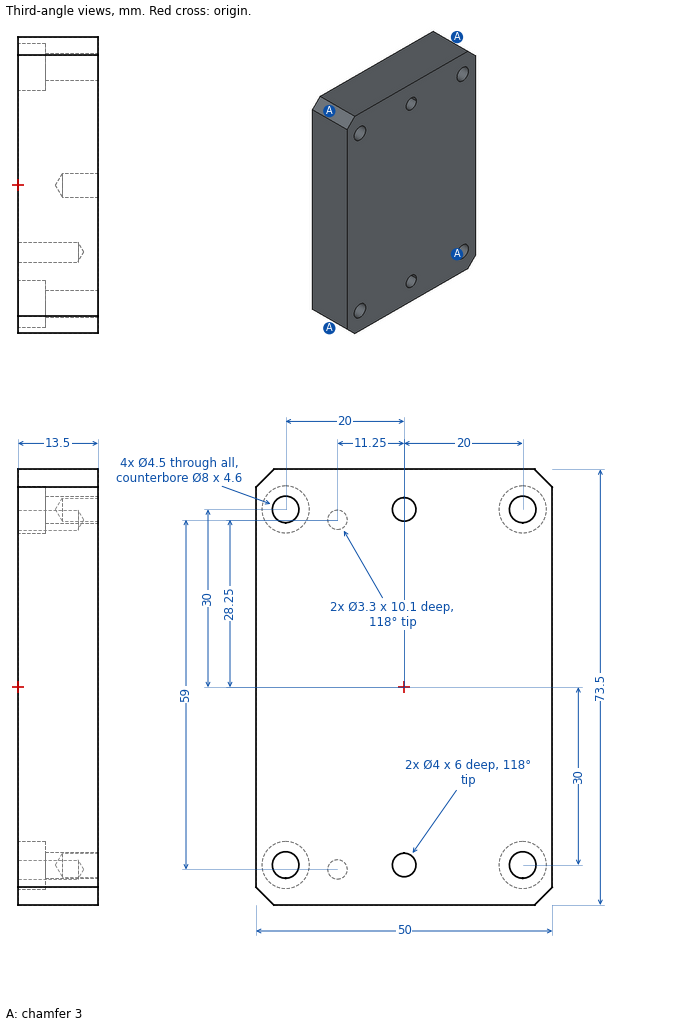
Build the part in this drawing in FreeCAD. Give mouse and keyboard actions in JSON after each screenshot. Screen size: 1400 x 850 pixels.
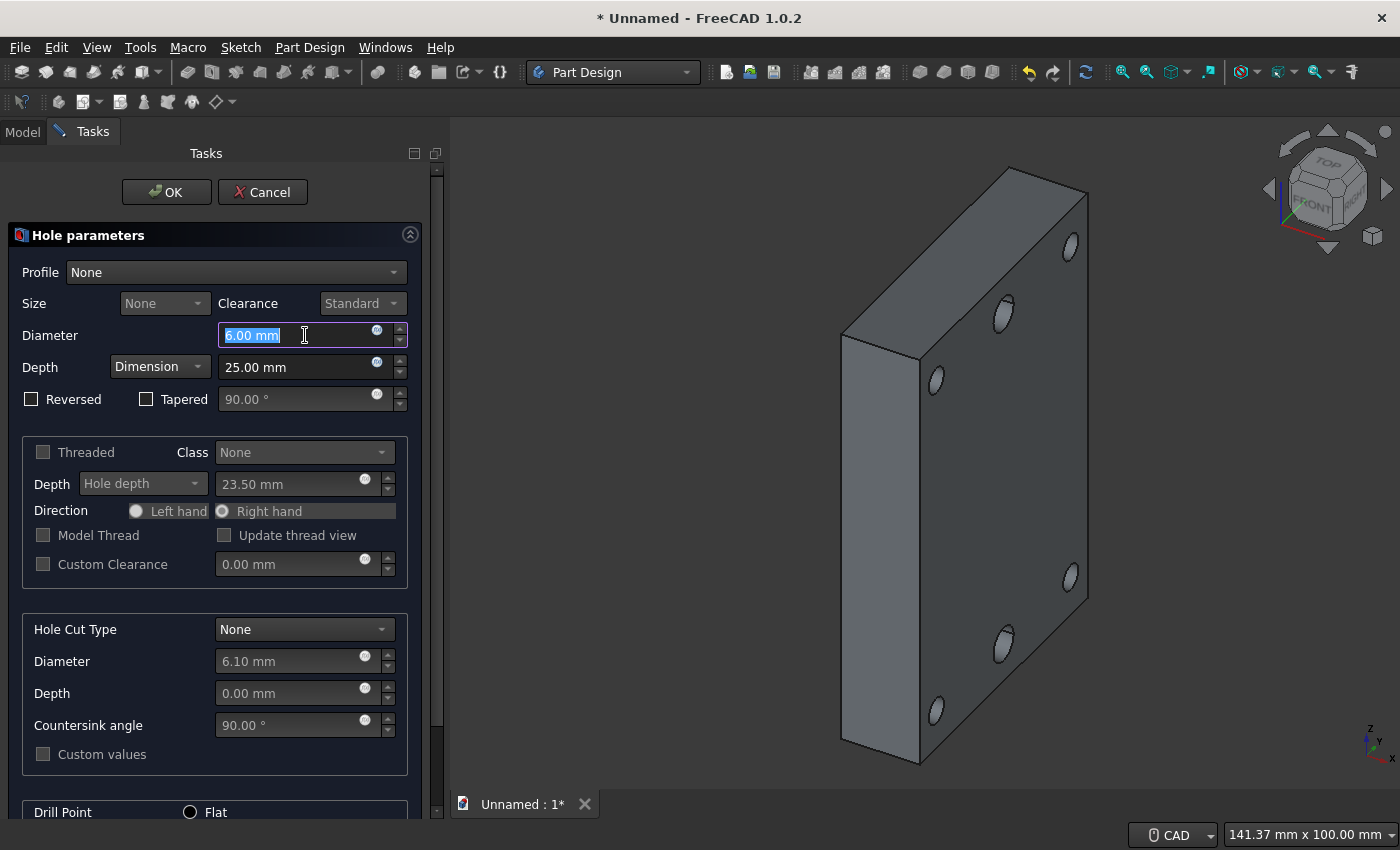
{"action": "type", "text": "4"}
{"action": "key", "text": "Tab"}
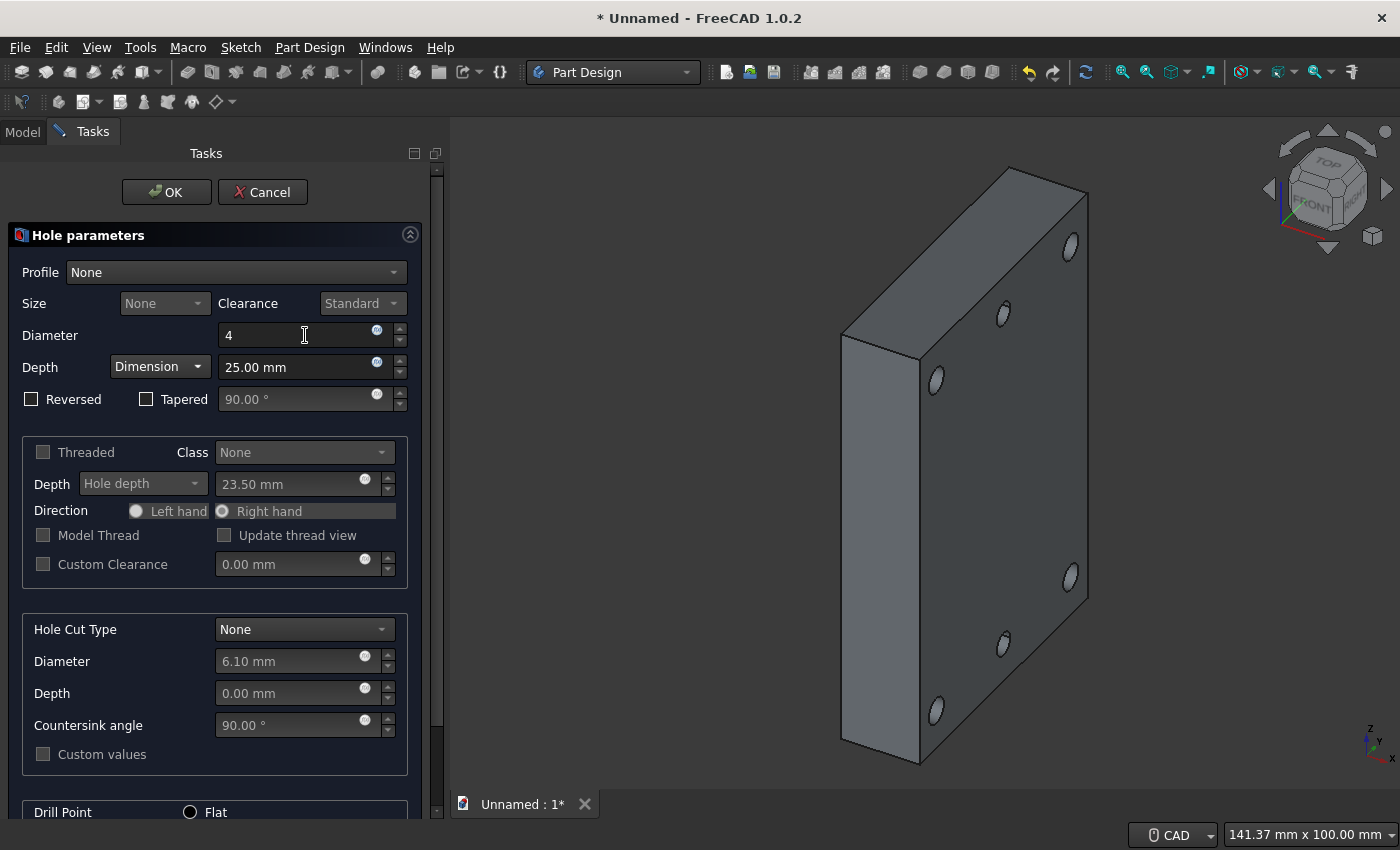
{"action": "triple_click", "coordinate": [305, 367]}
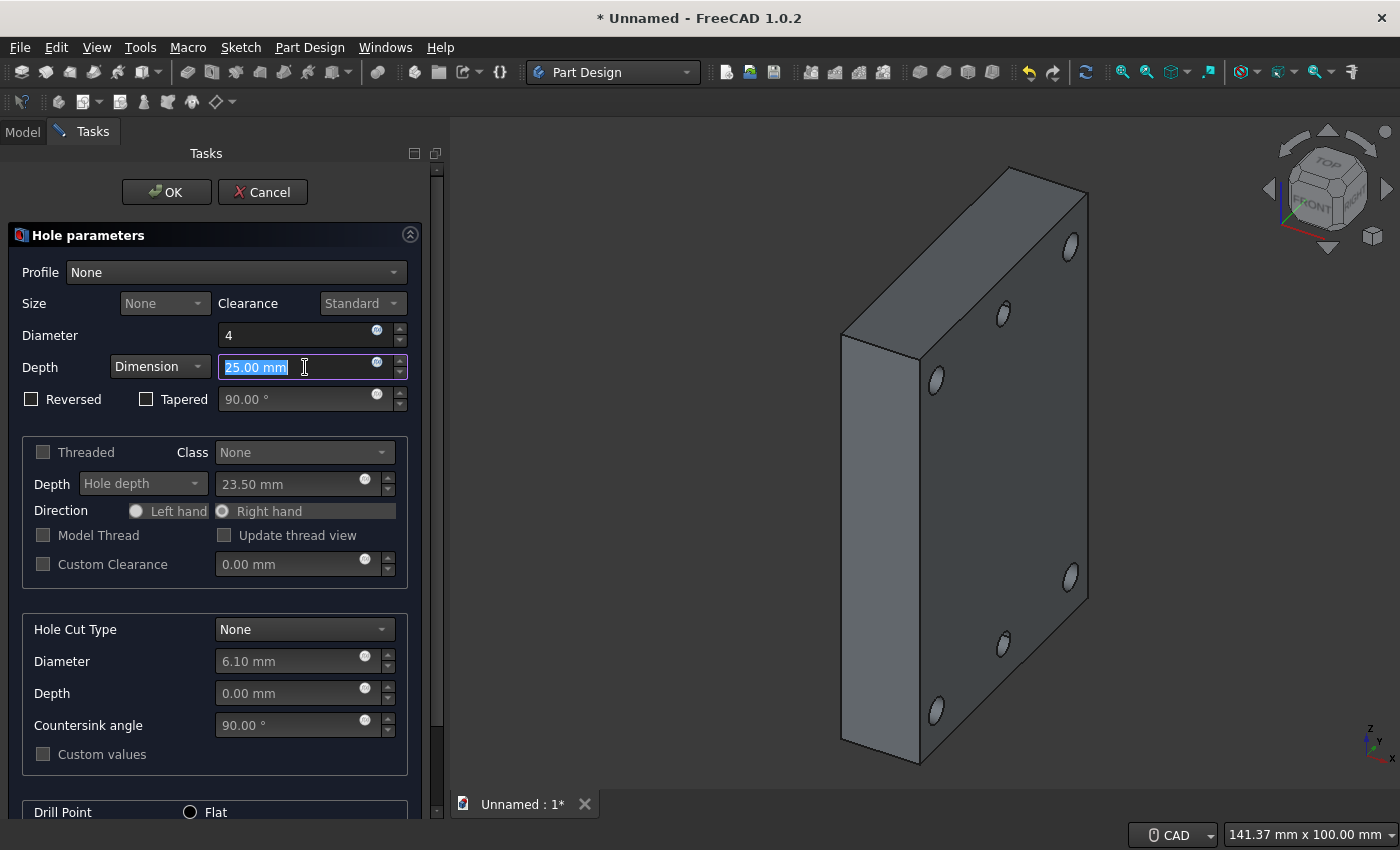
{"action": "type", "text": "6"}
{"action": "key", "text": "Tab"}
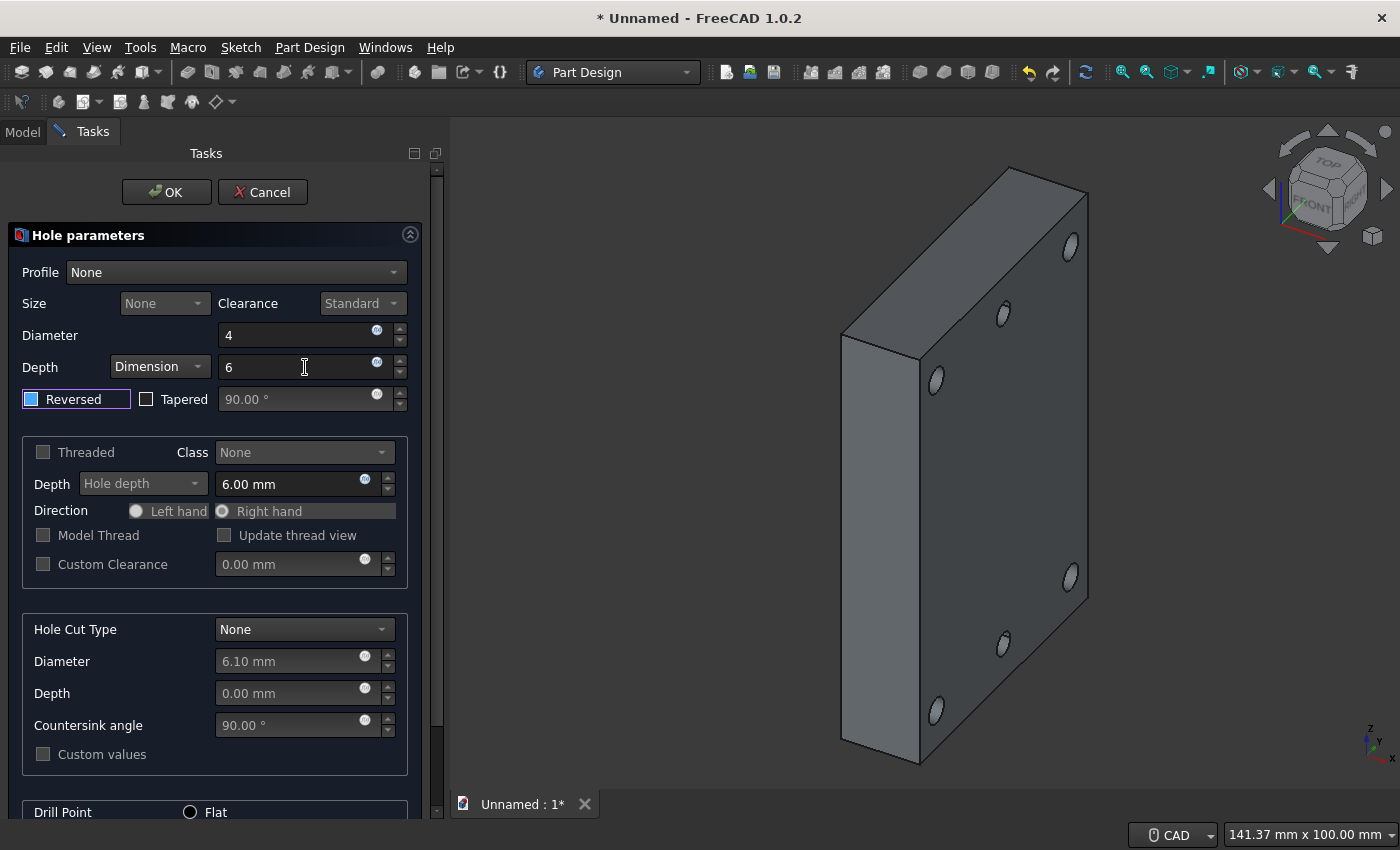
{"action": "left_click", "coordinate": [167, 192]}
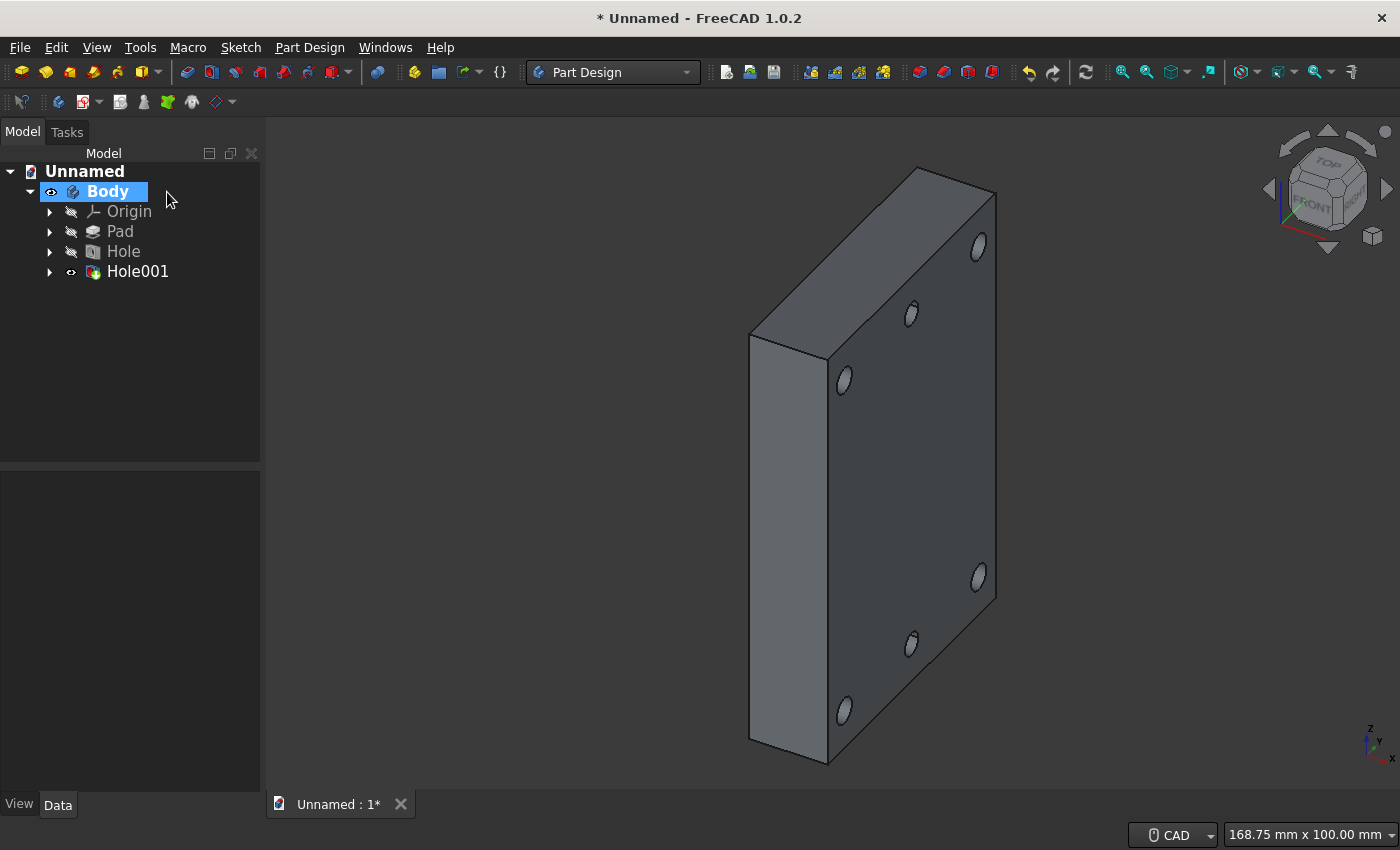
{"action": "key", "text": "6"}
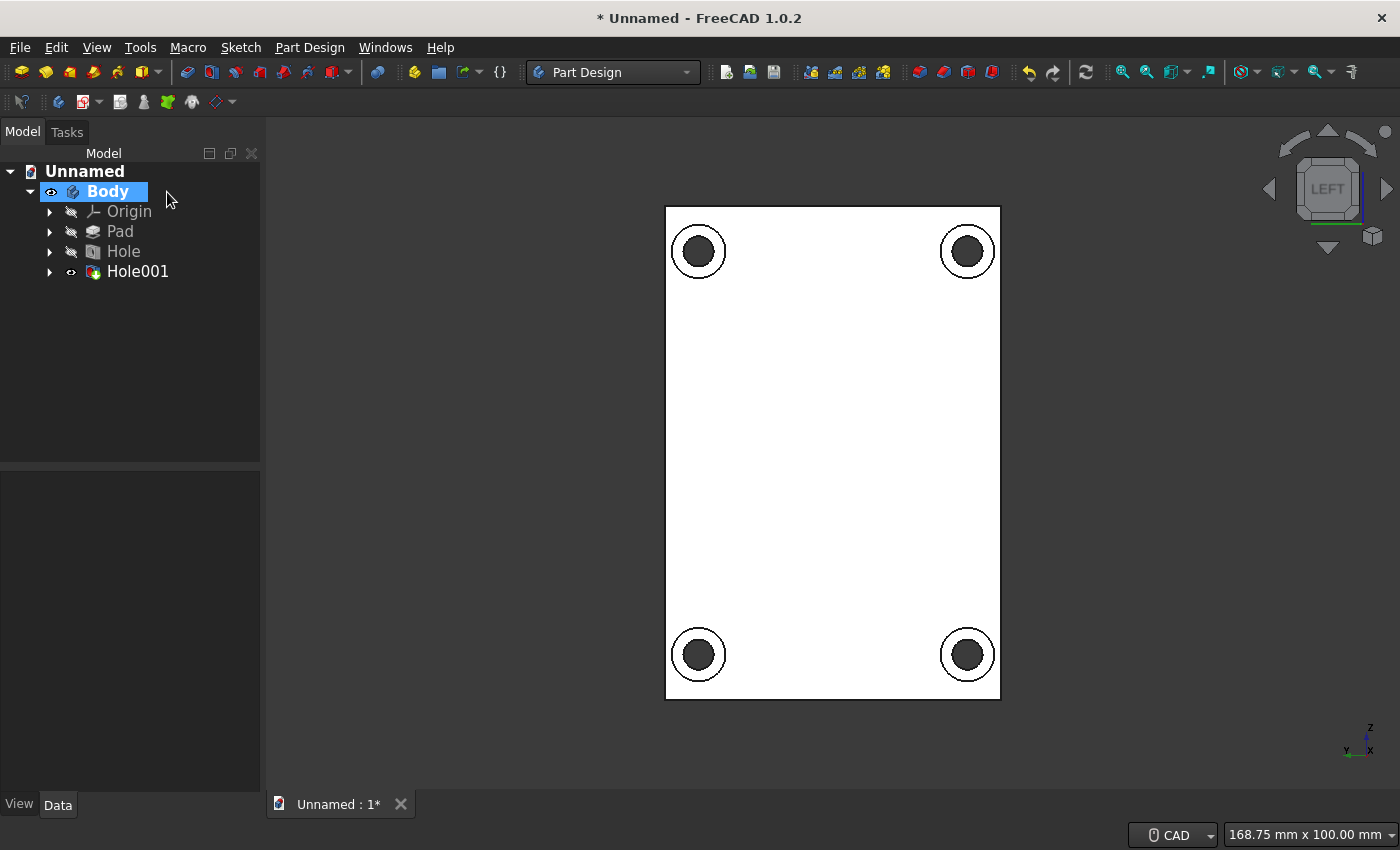
{"action": "left_click", "coordinate": [833, 452]}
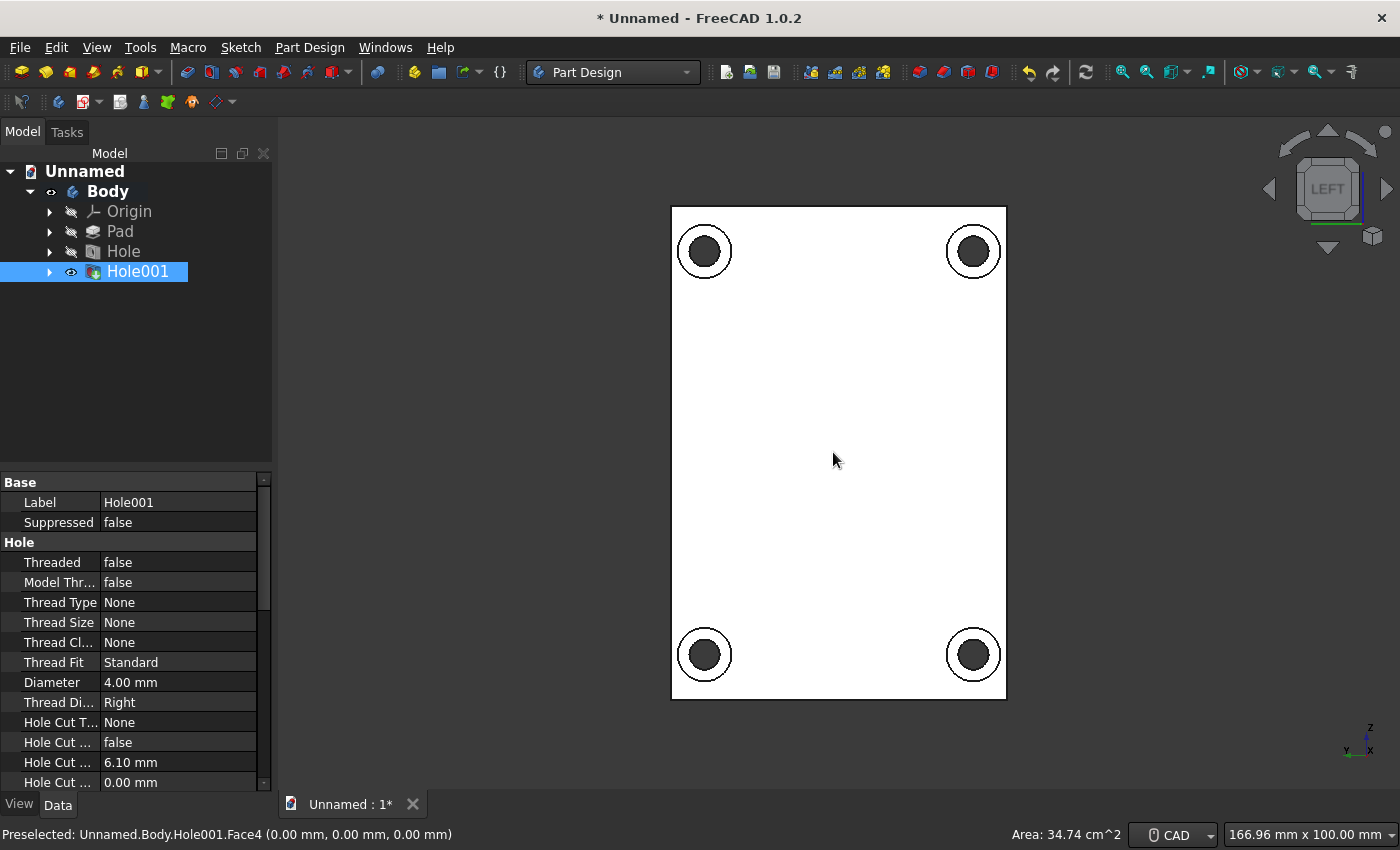
{"action": "left_click", "coordinate": [84, 102]}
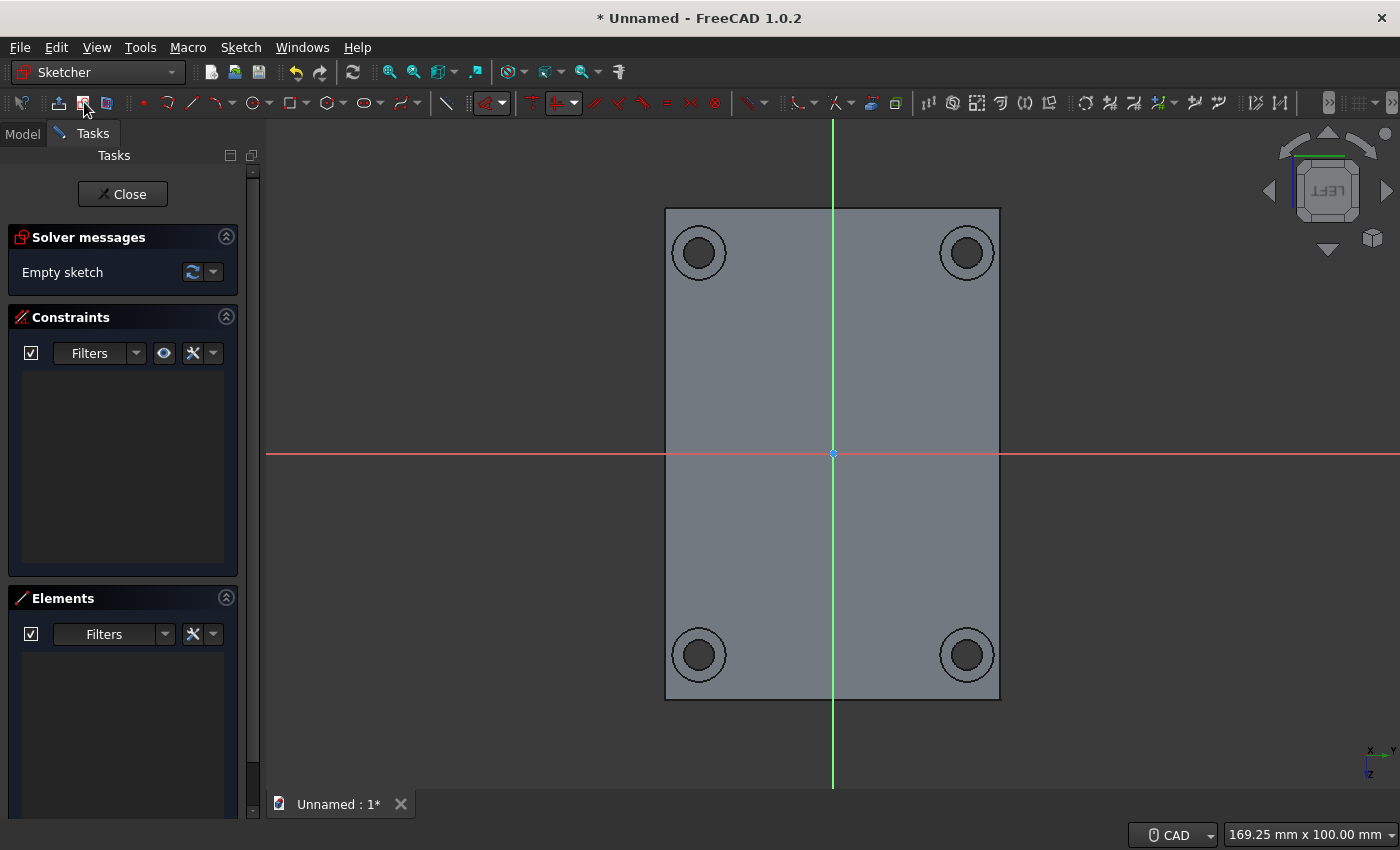
{"action": "left_click", "coordinate": [254, 104]}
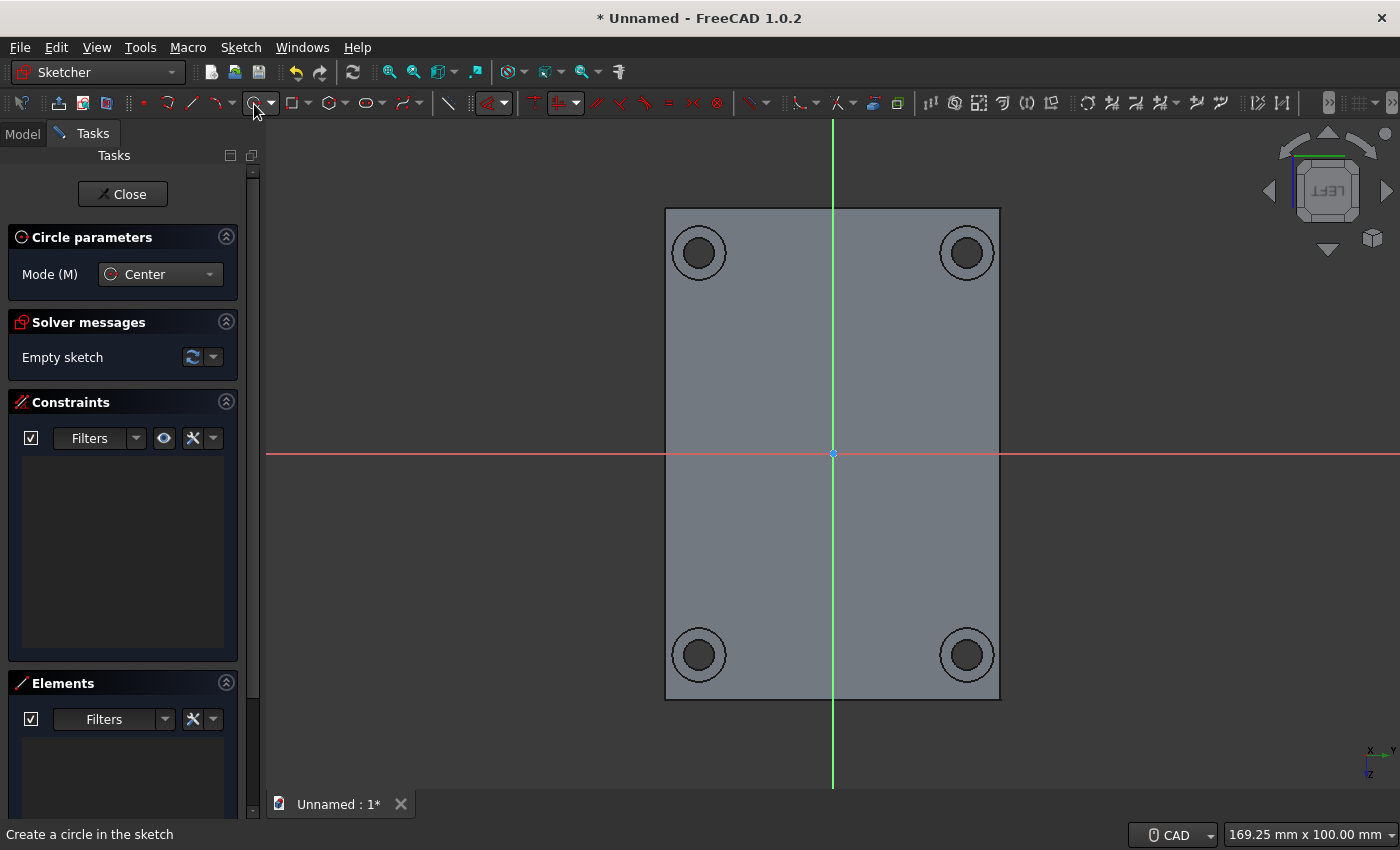
{"action": "scroll", "coordinate": [758, 643], "scroll_direction": "up", "scroll_amount": 4}